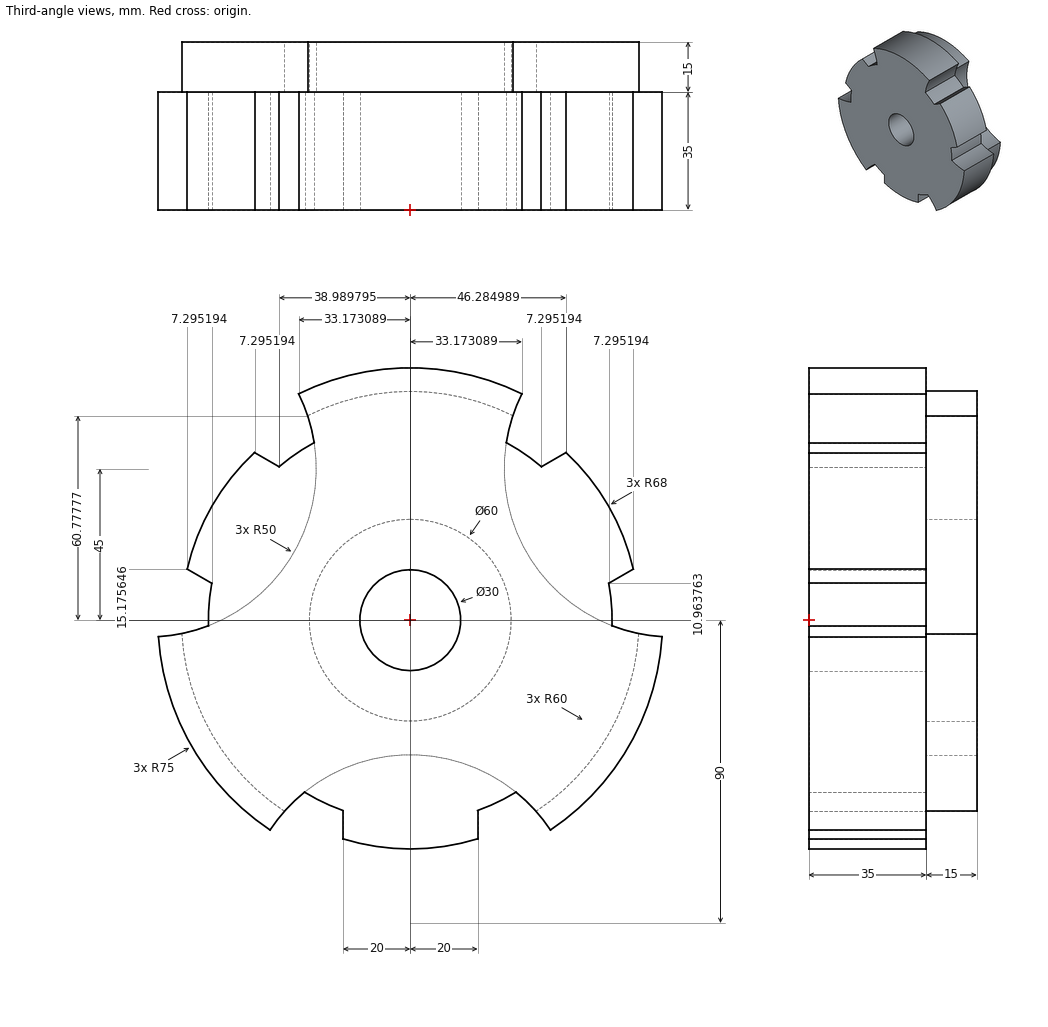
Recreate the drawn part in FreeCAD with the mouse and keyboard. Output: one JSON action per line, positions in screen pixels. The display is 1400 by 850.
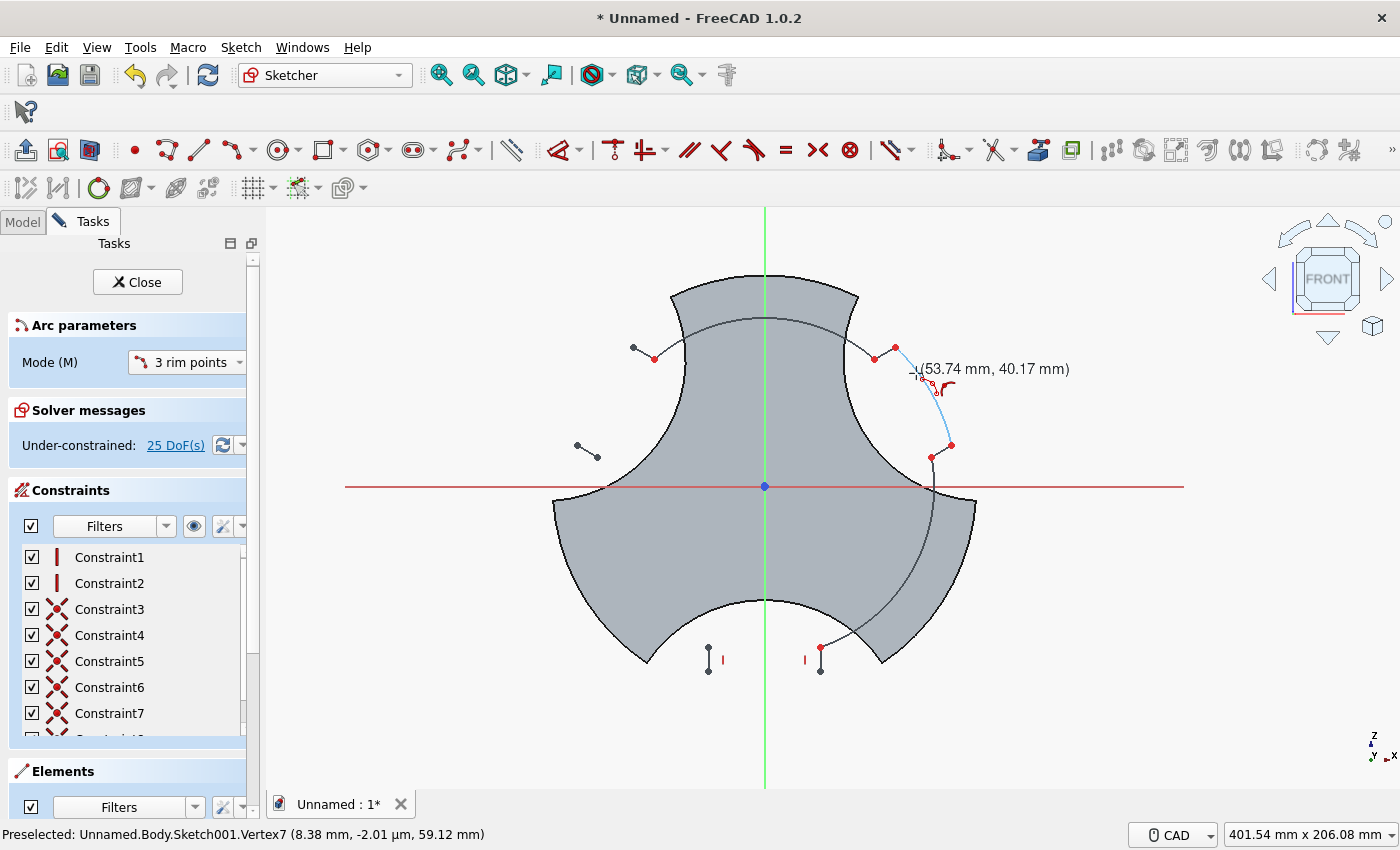
{"action": "scroll", "coordinate": [634, 346], "scroll_direction": "up", "scroll_amount": 2}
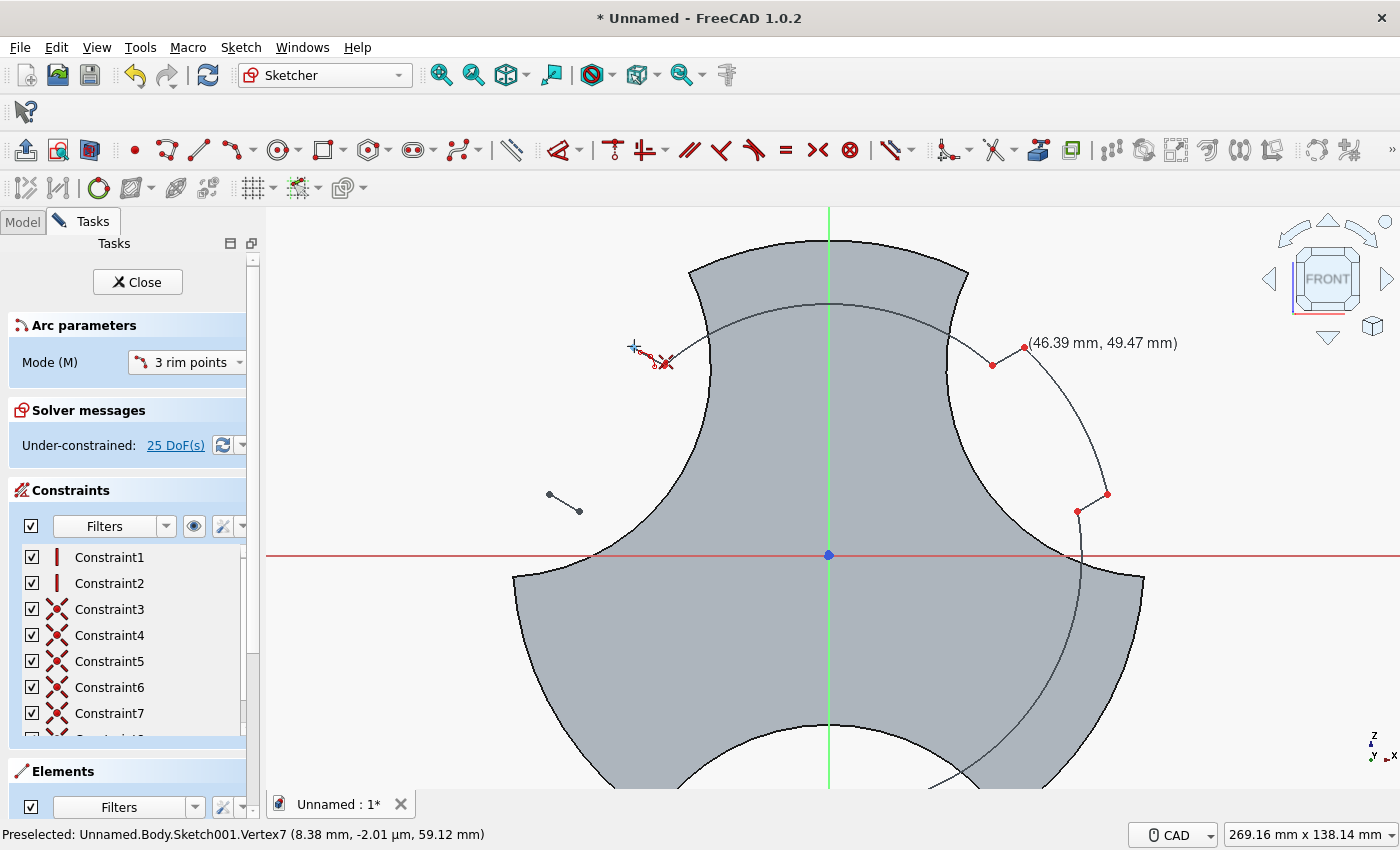
{"action": "left_click", "coordinate": [633, 348]}
{"action": "left_click", "coordinate": [550, 494]}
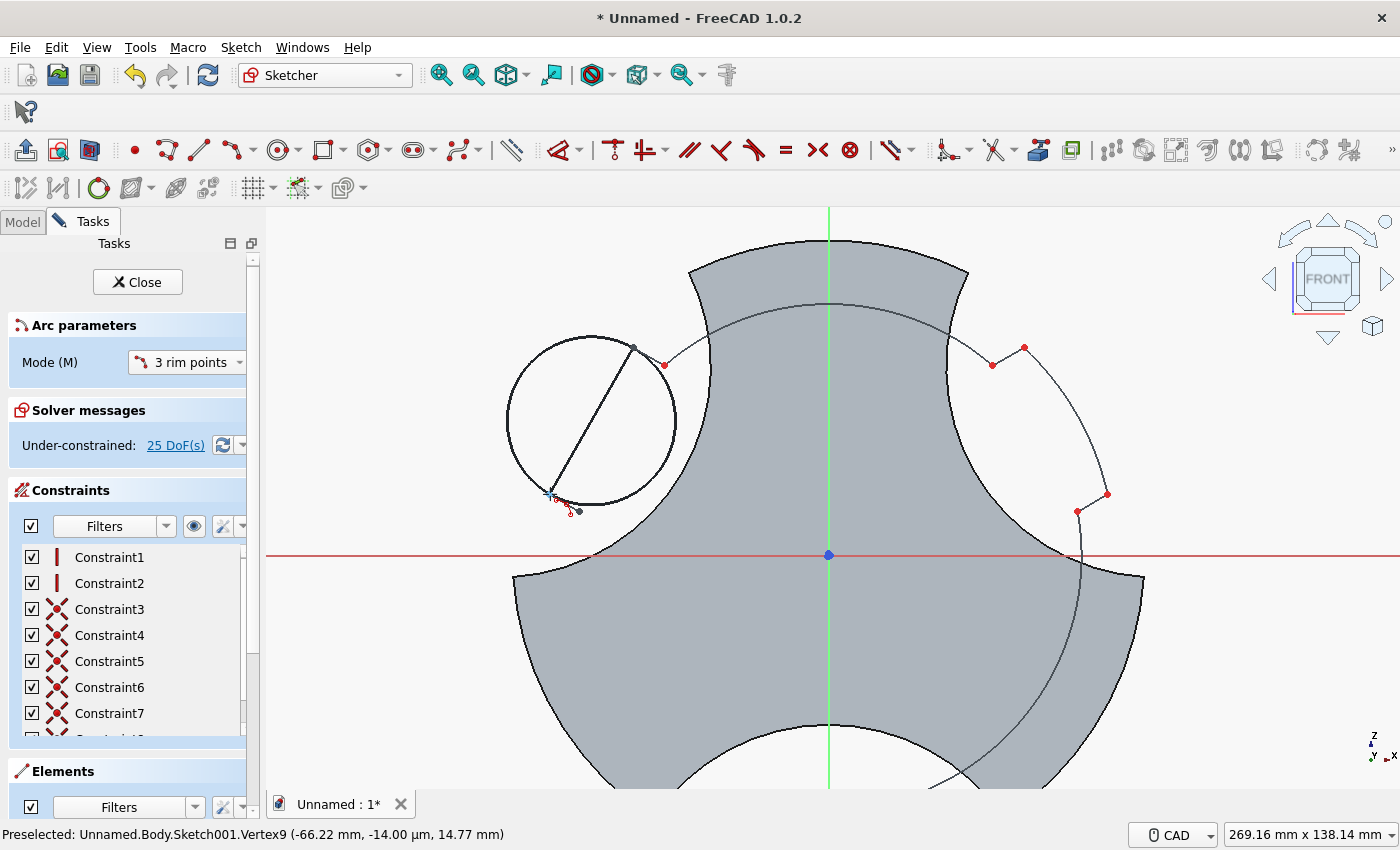
{"action": "scroll", "coordinate": [580, 413], "scroll_direction": "up", "scroll_amount": 2}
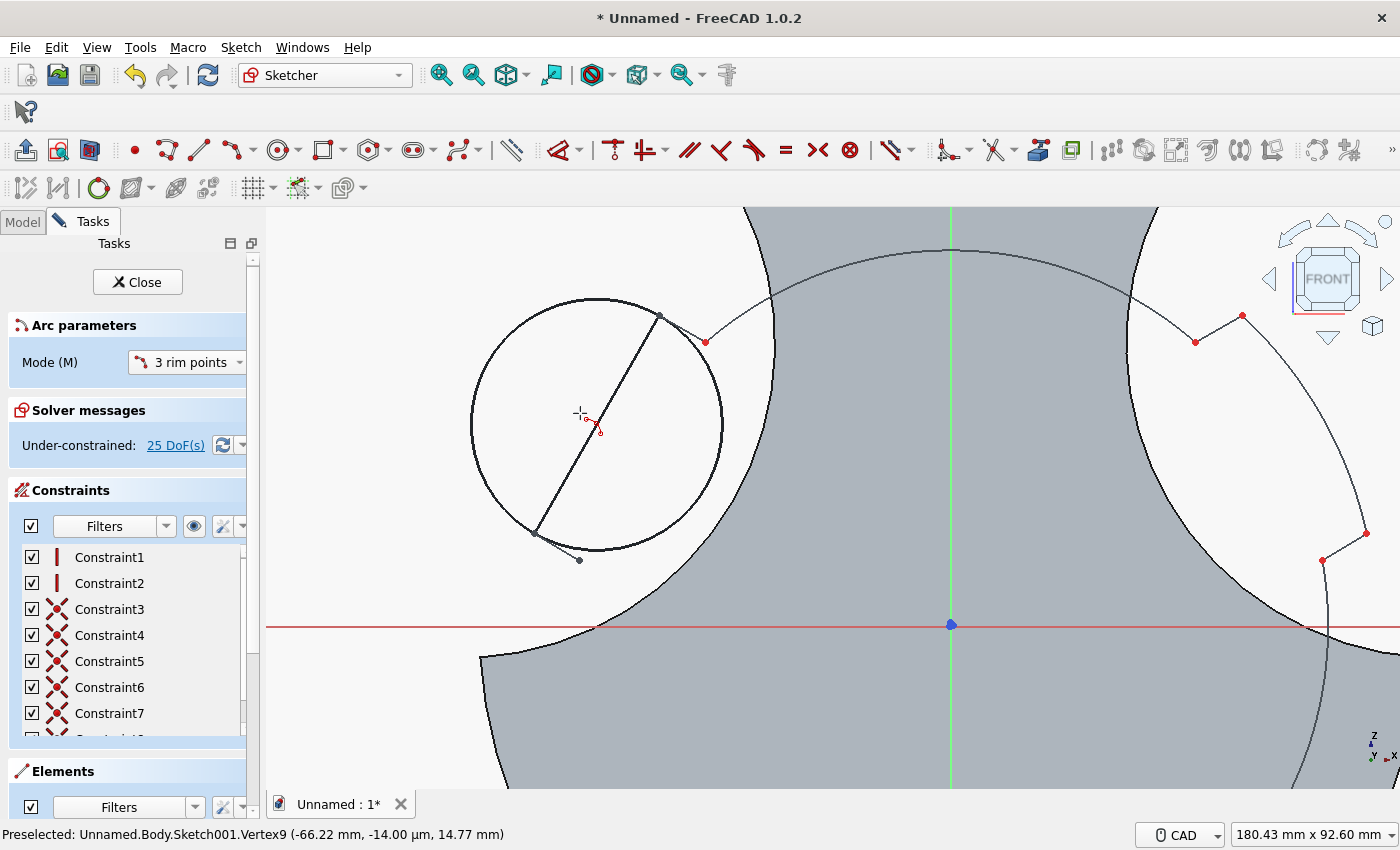
{"action": "left_click", "coordinate": [581, 413]}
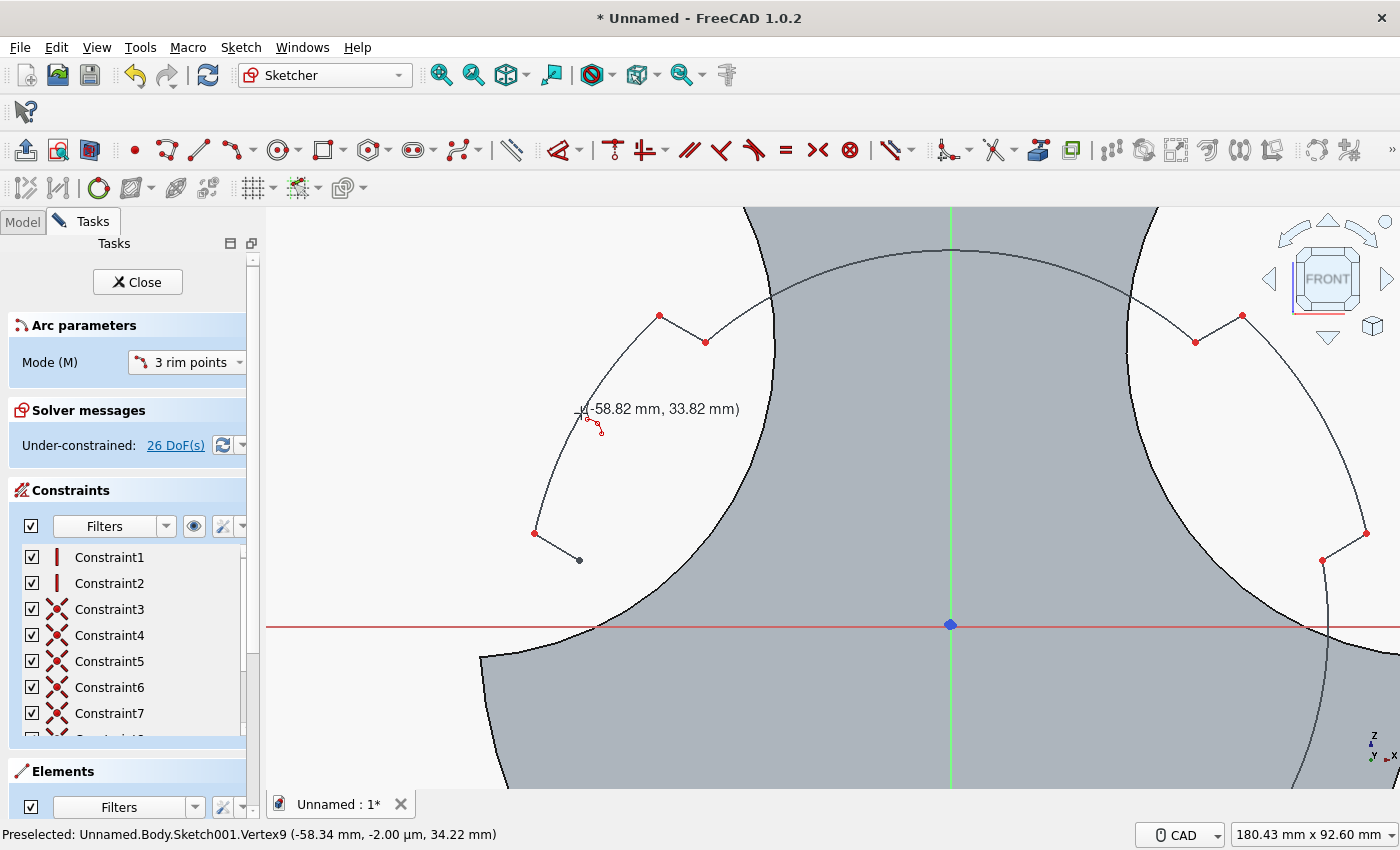
{"action": "left_click", "coordinate": [579, 560]}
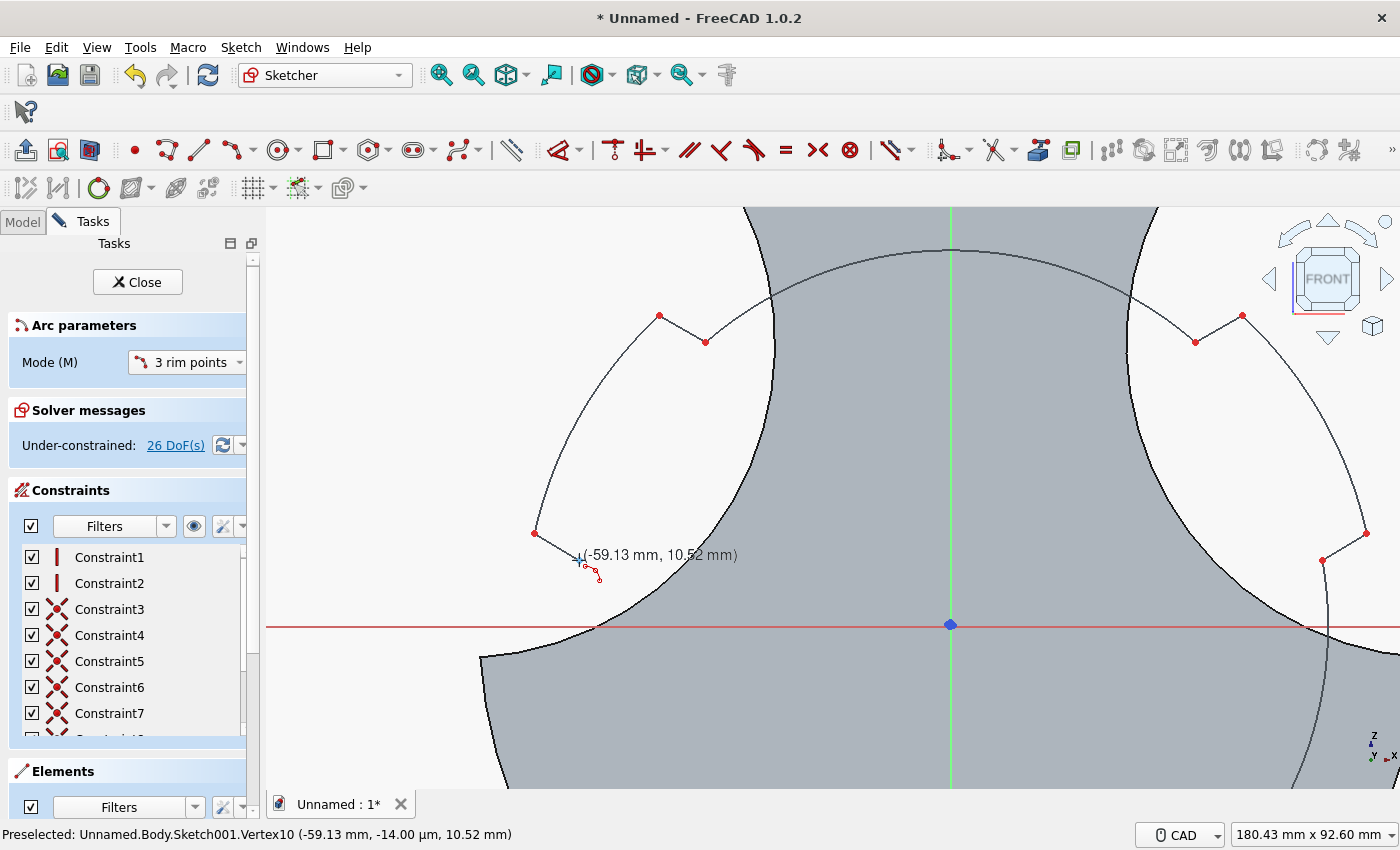
{"action": "scroll", "coordinate": [613, 373], "scroll_direction": "down", "scroll_amount": 4}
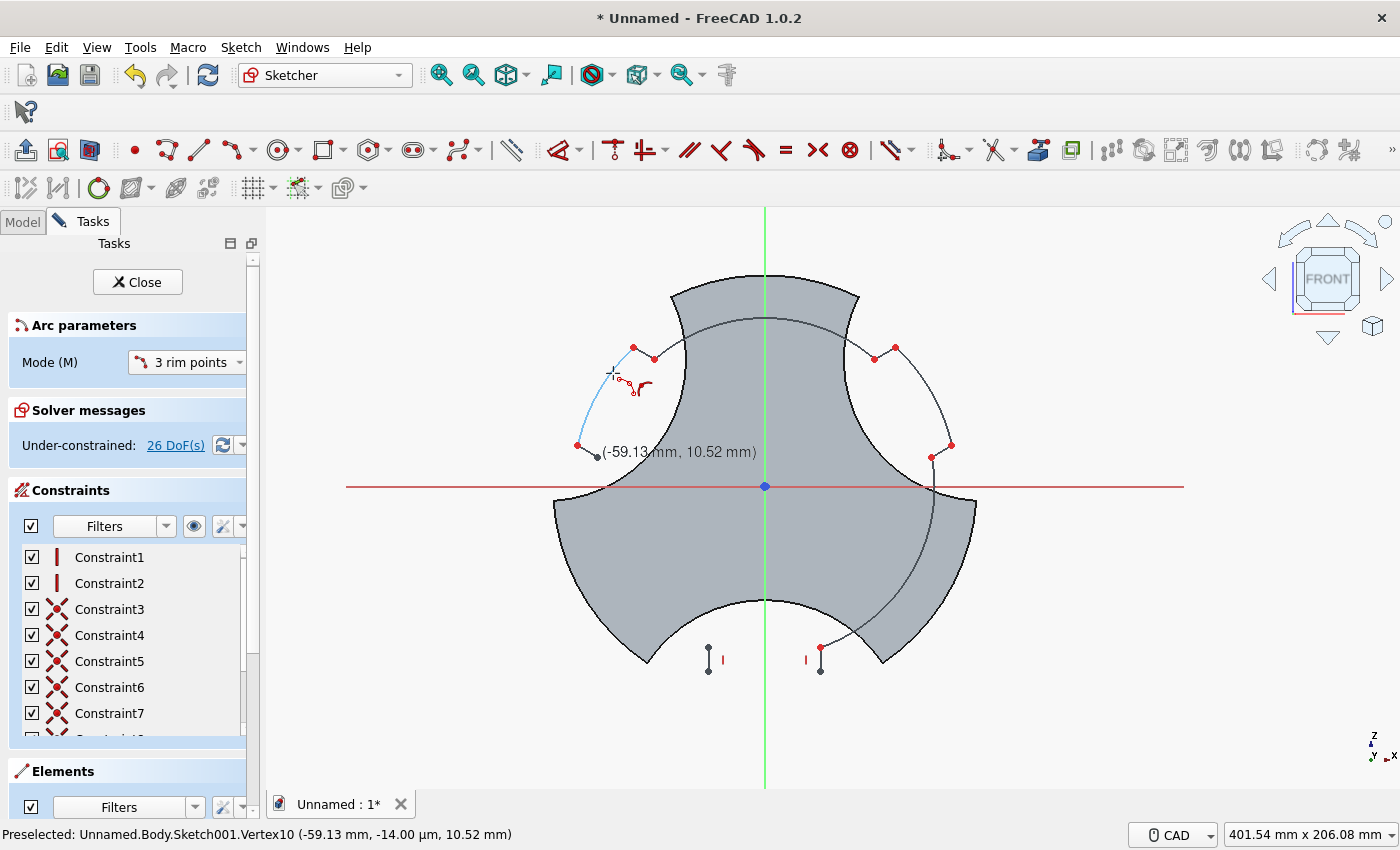
{"action": "scroll", "coordinate": [708, 647], "scroll_direction": "up", "scroll_amount": 2}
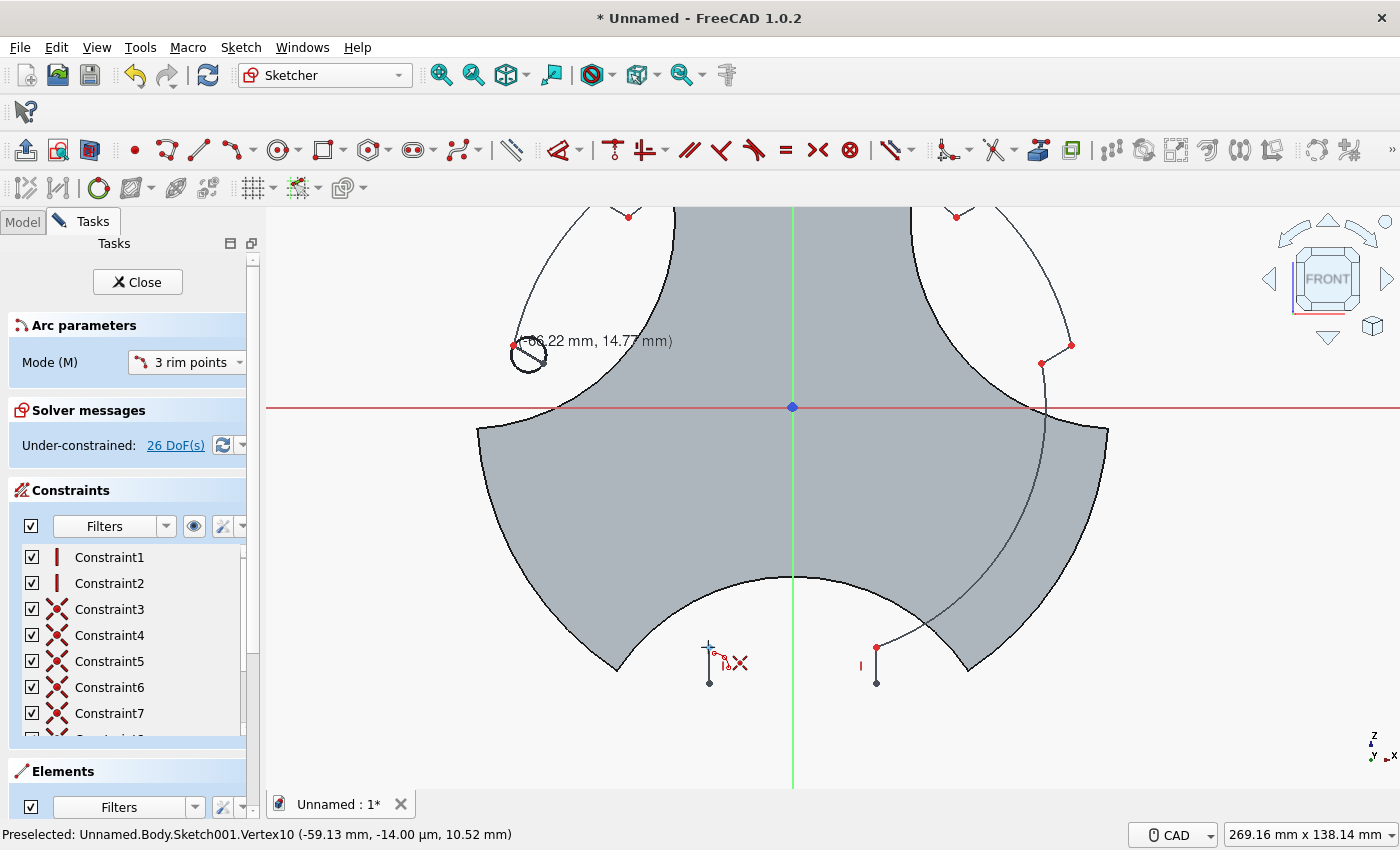
{"action": "left_click", "coordinate": [709, 647]}
{"action": "left_click", "coordinate": [574, 534]}